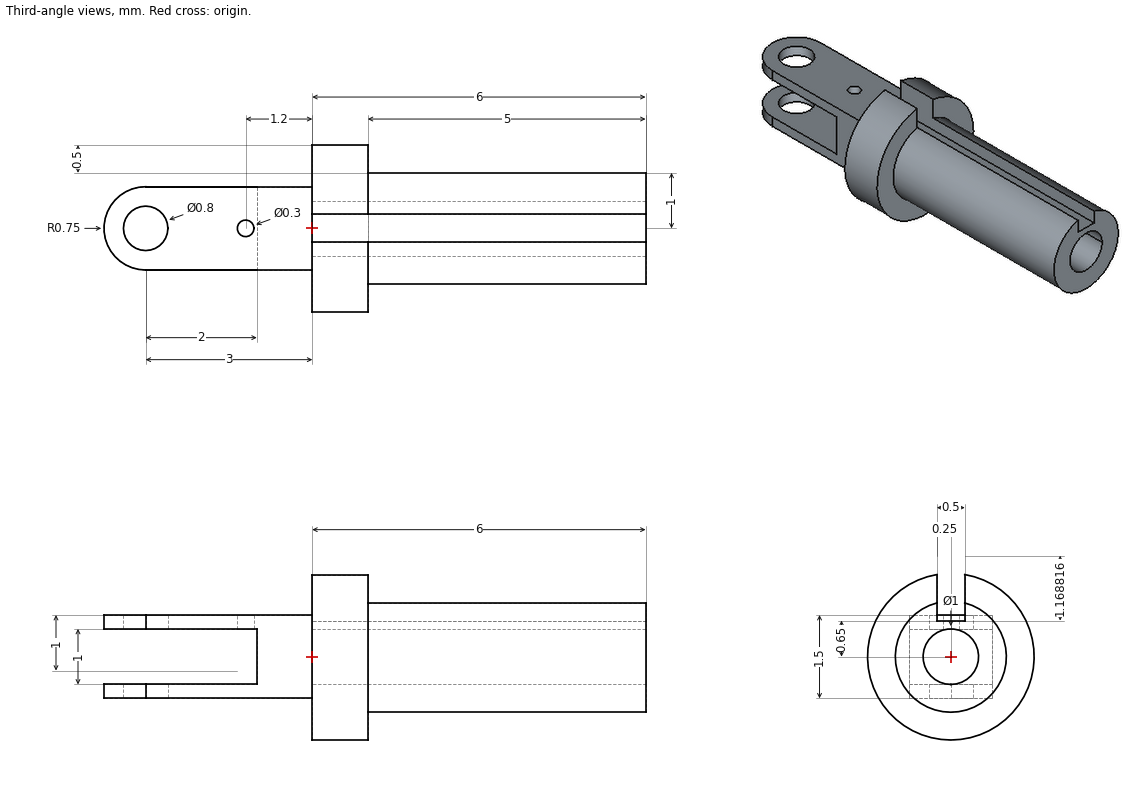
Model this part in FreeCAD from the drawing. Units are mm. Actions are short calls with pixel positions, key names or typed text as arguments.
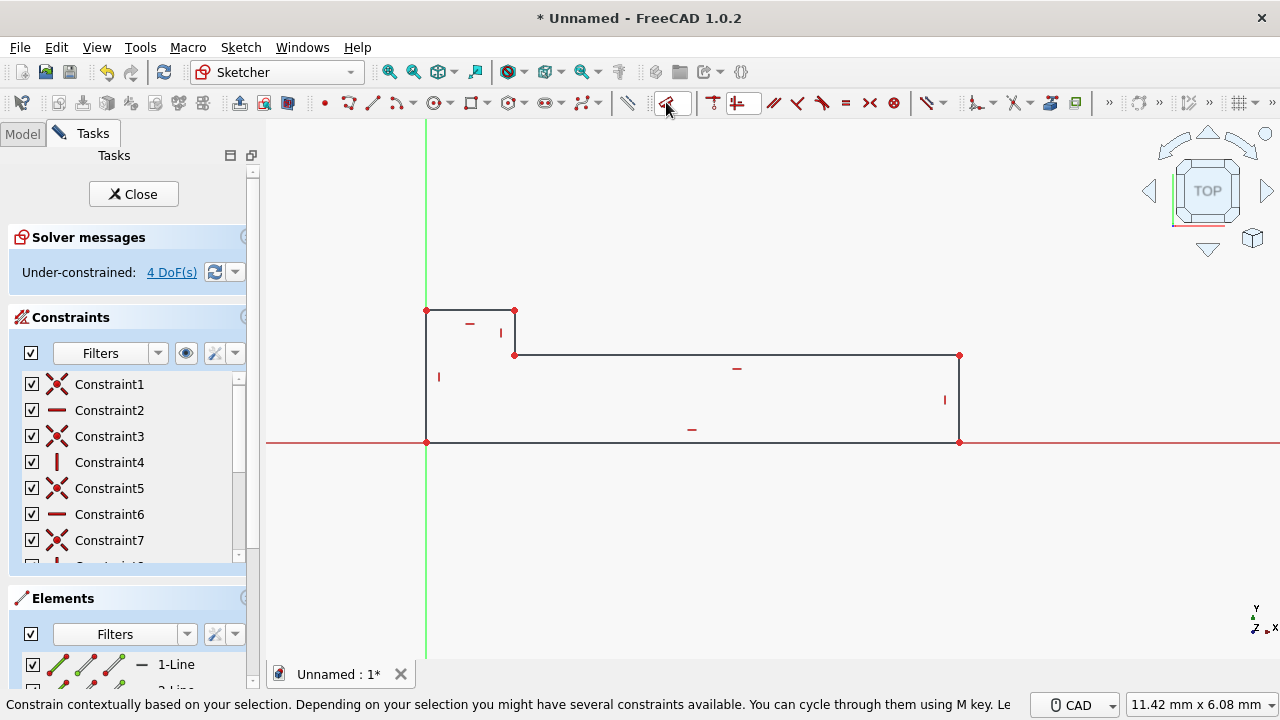
click(586, 443)
click(693, 477)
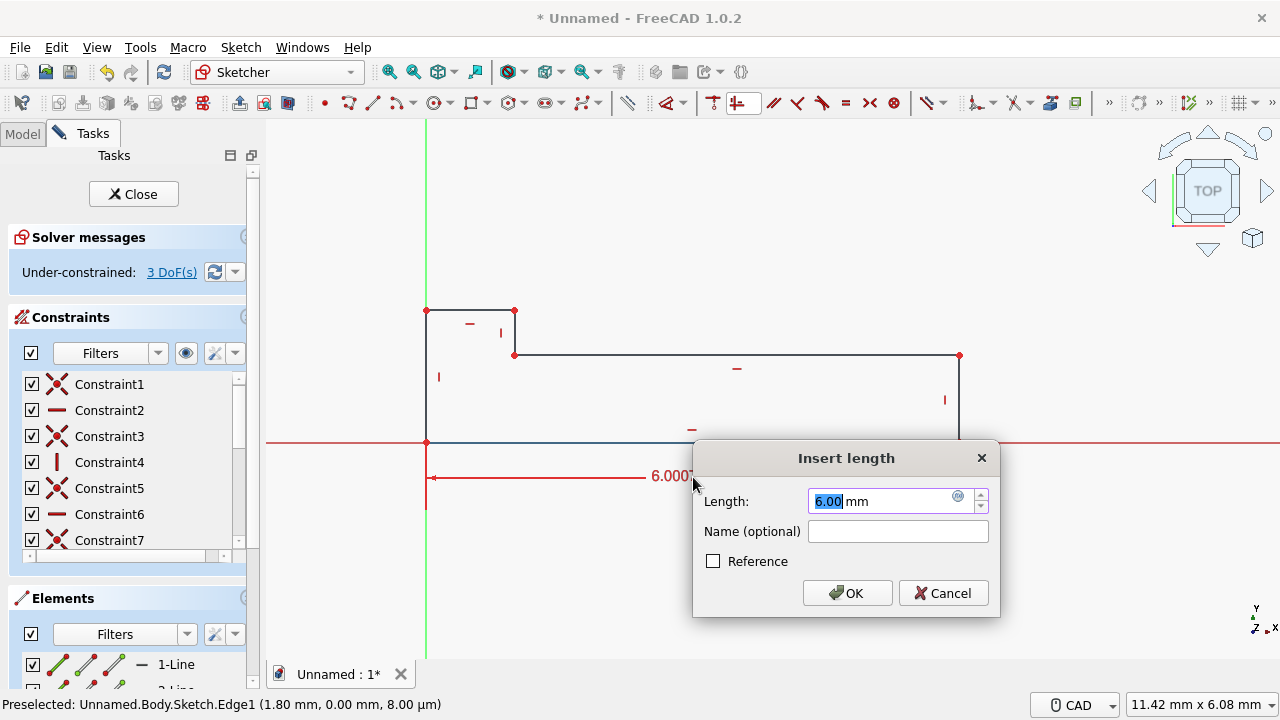
text(6)
key(Return)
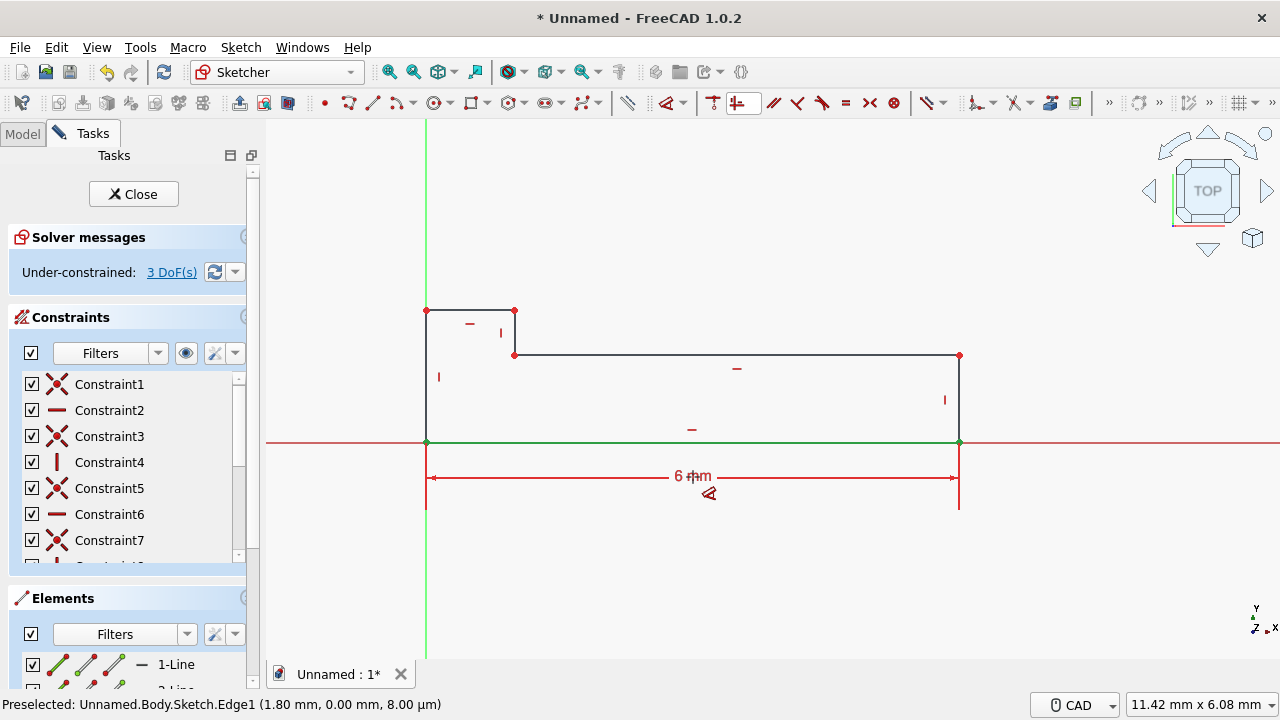
click(959, 417)
click(993, 399)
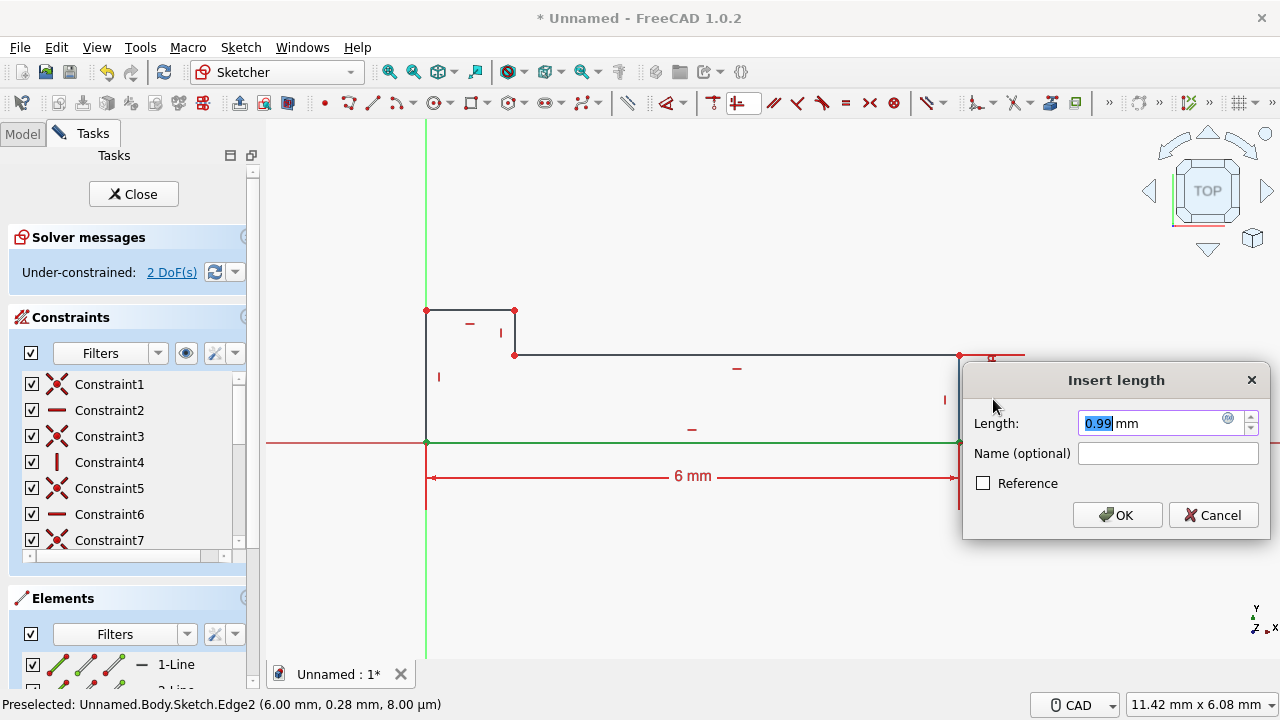
text(1)
key(Return)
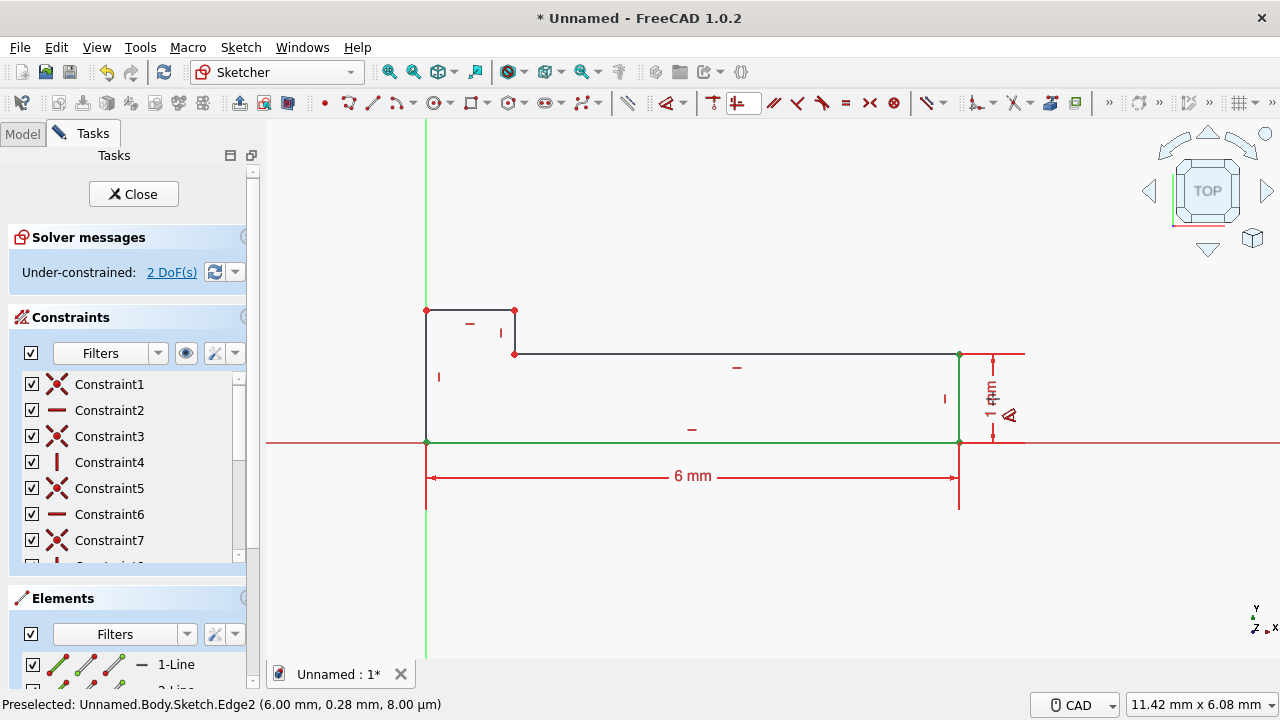
click(826, 354)
click(737, 320)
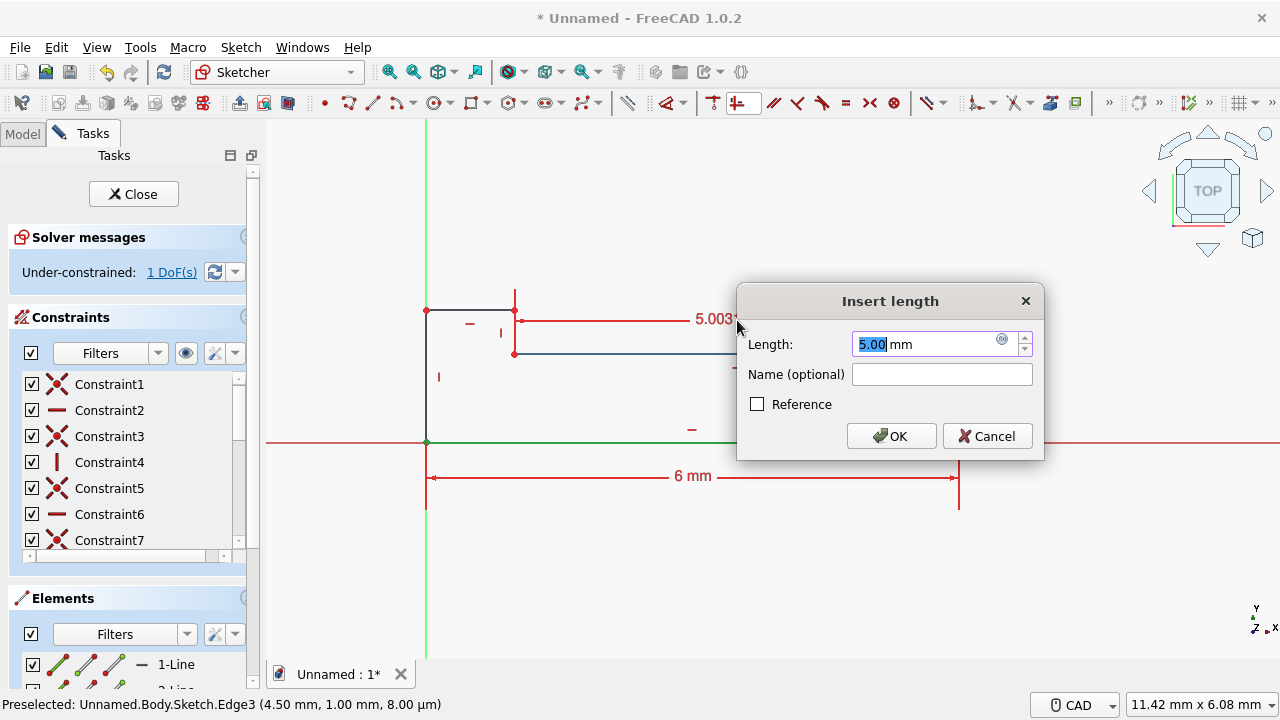
text(5)
key(Return)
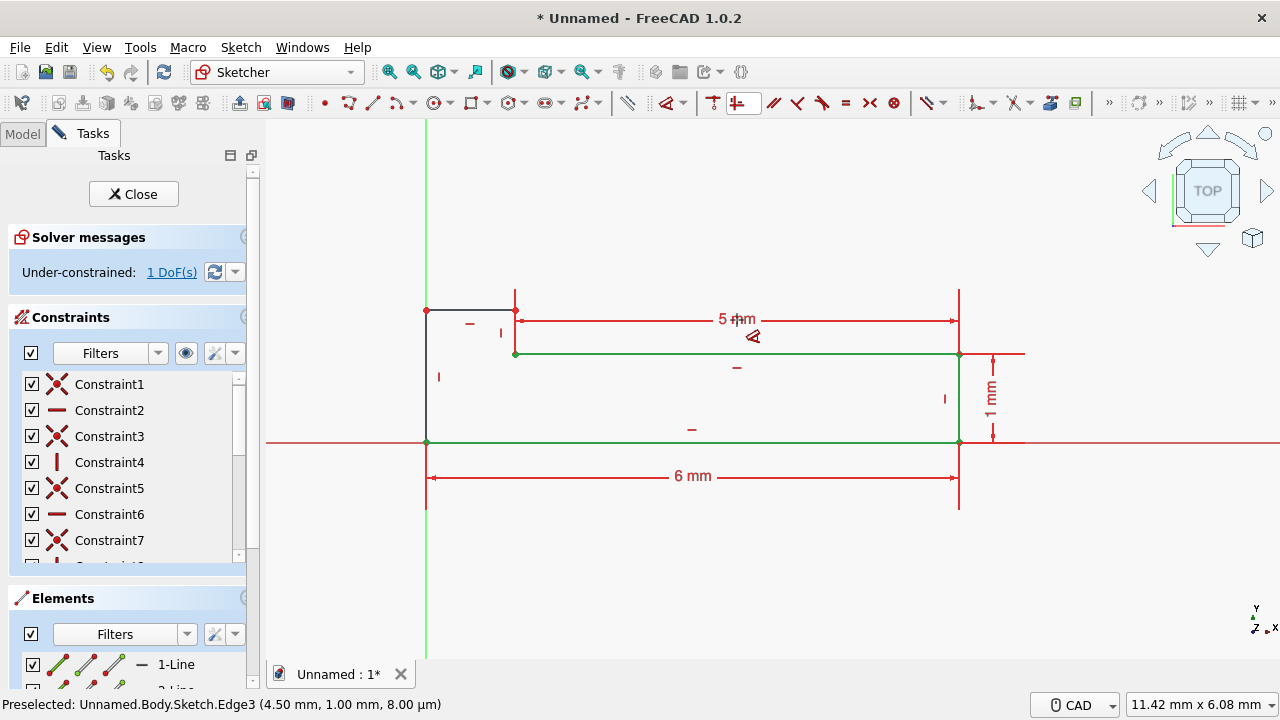
click(515, 341)
click(481, 332)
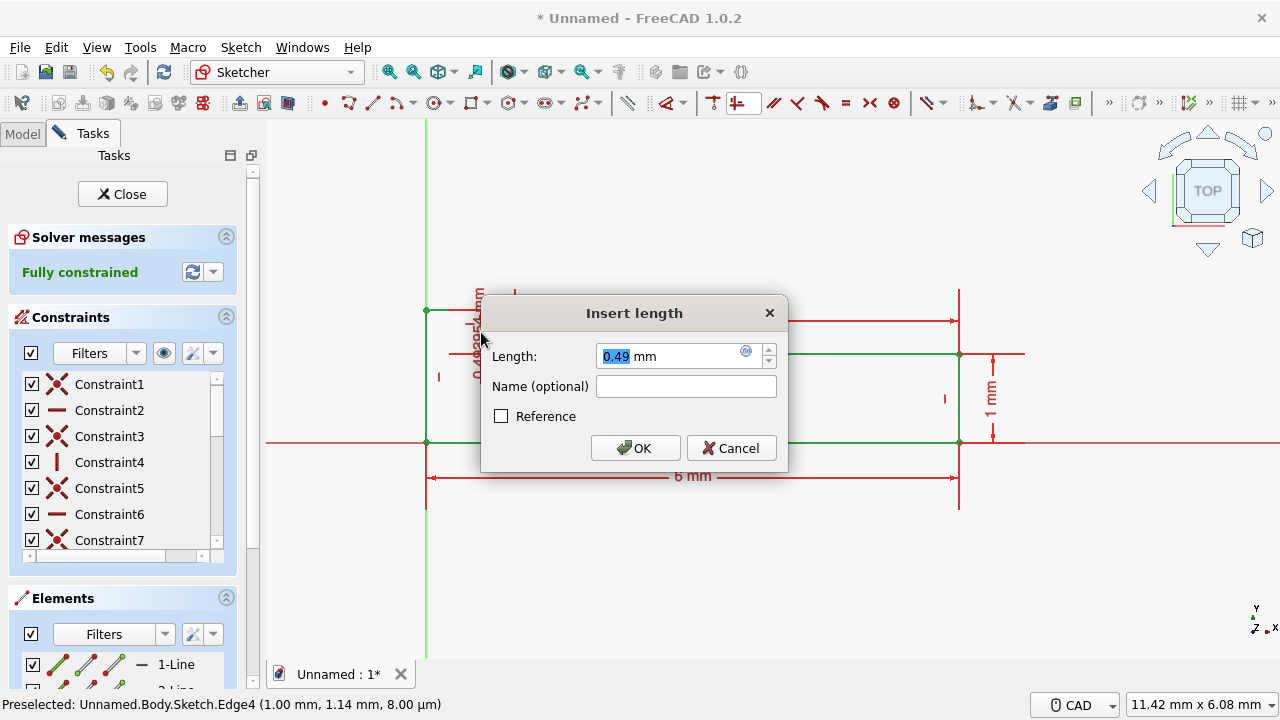
text(0.5)
key(Return)
key(Escape)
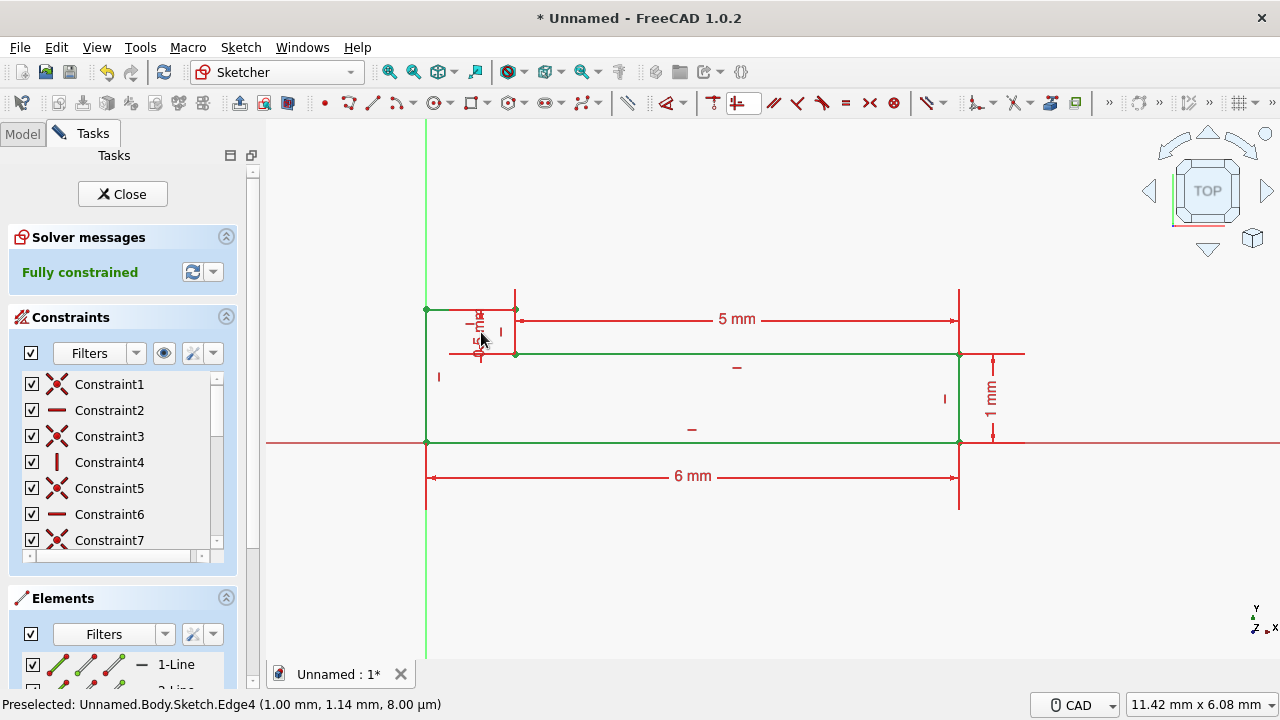
click(123, 194)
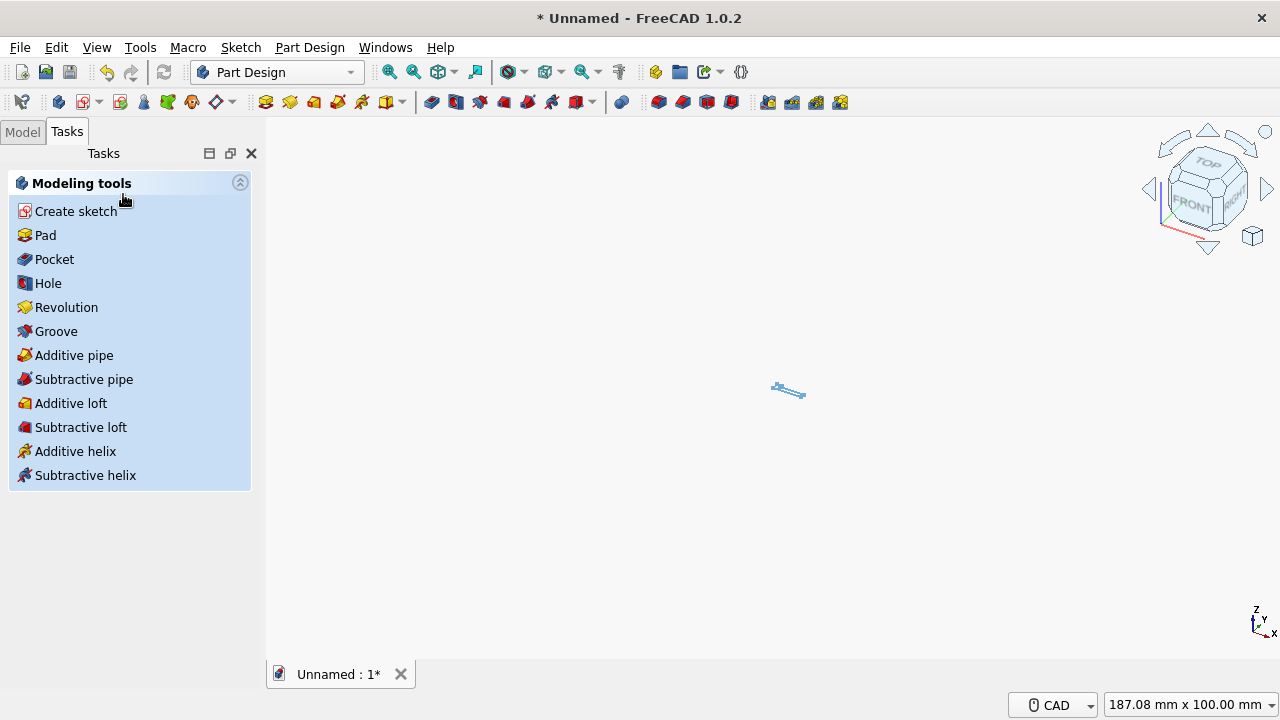
click(290, 102)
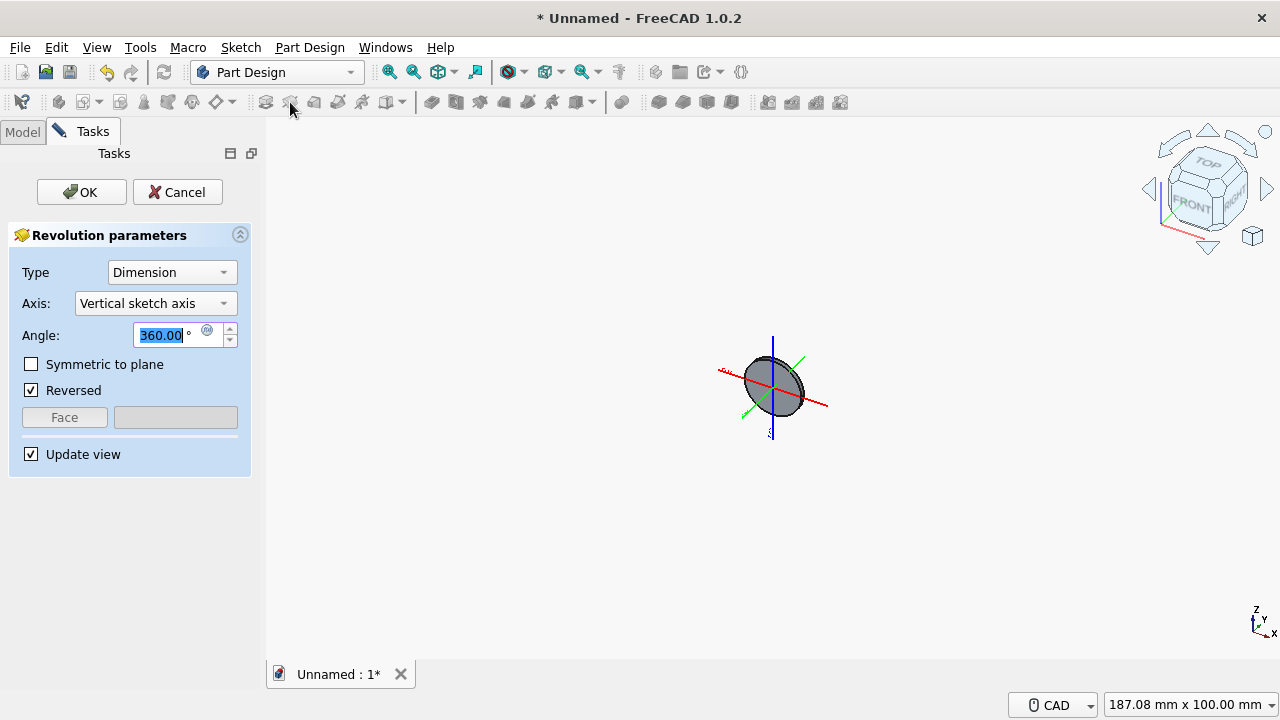
click(156, 304)